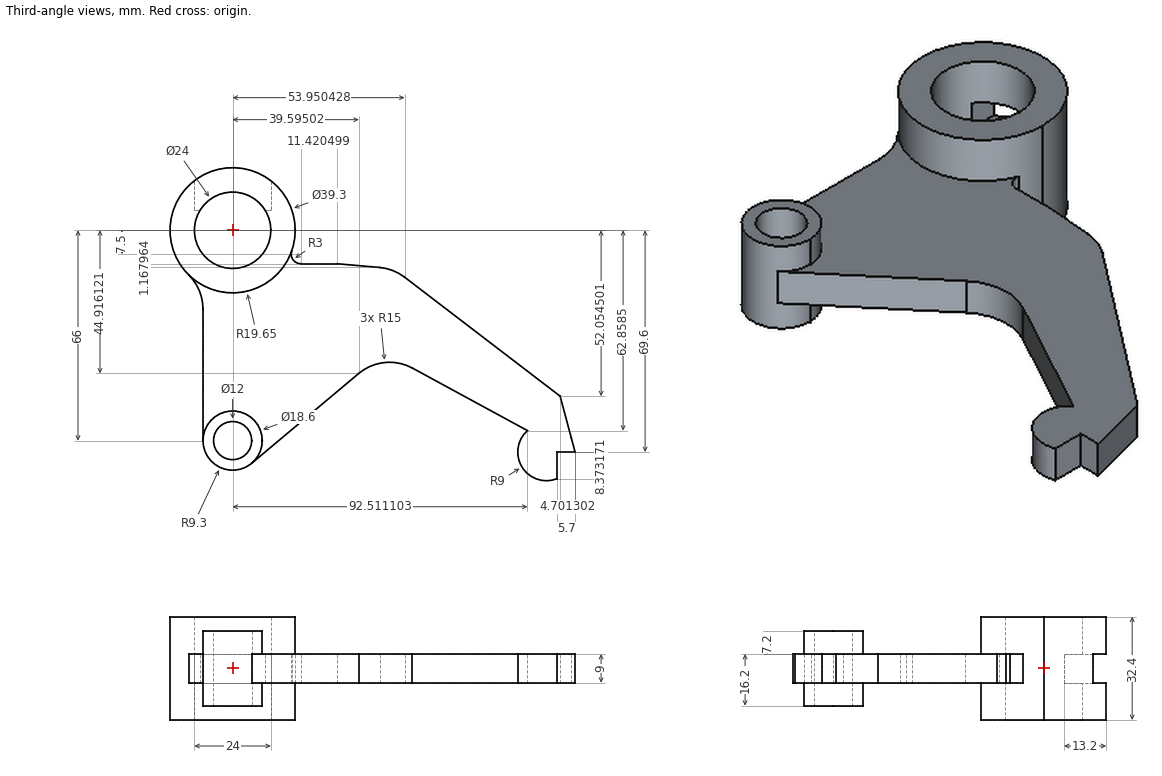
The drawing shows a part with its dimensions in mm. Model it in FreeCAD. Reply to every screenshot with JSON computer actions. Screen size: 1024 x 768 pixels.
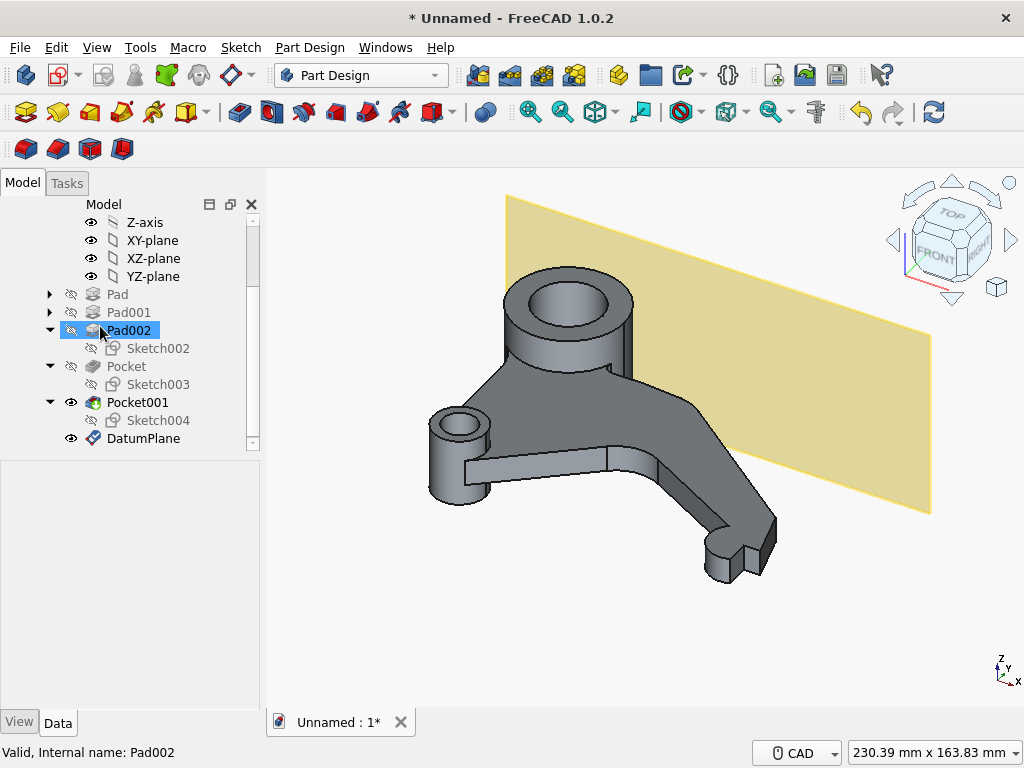
{"action": "left_click", "coordinate": [116, 438]}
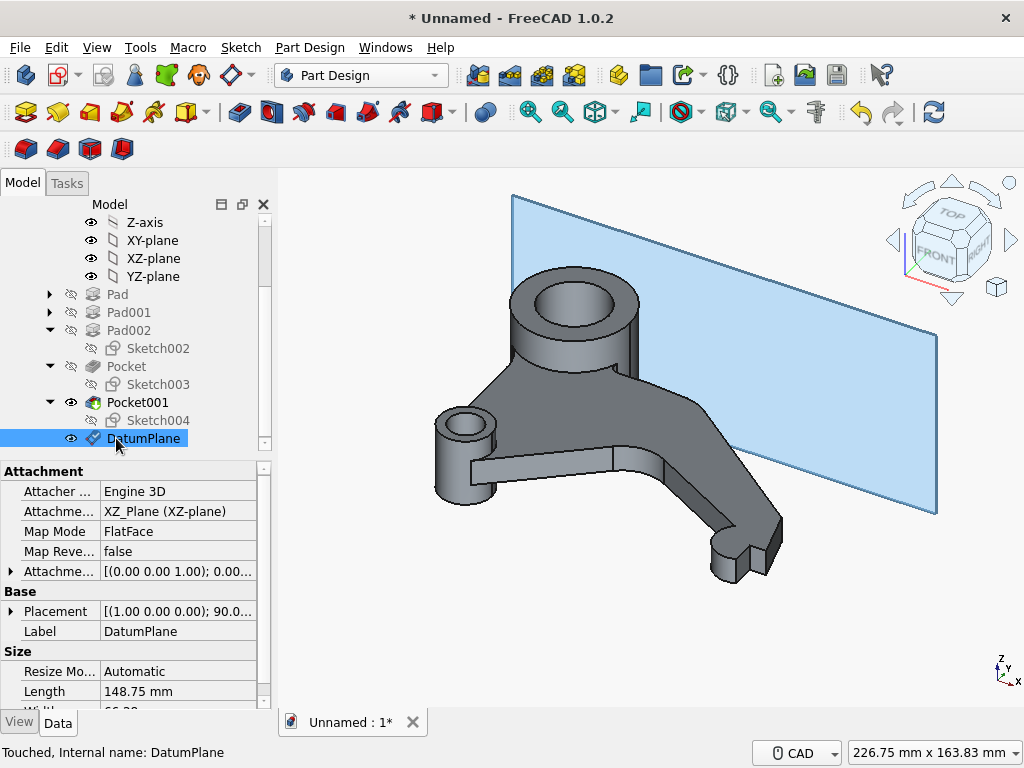
{"action": "left_click", "coordinate": [58, 76]}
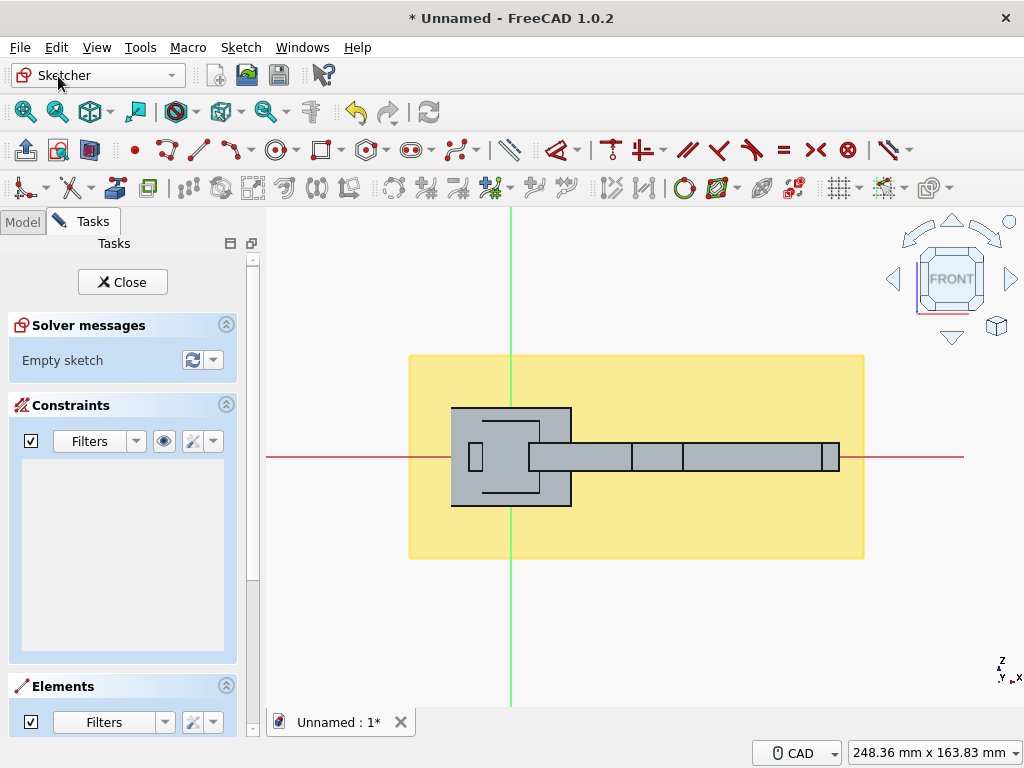
{"action": "key", "text": "q s"}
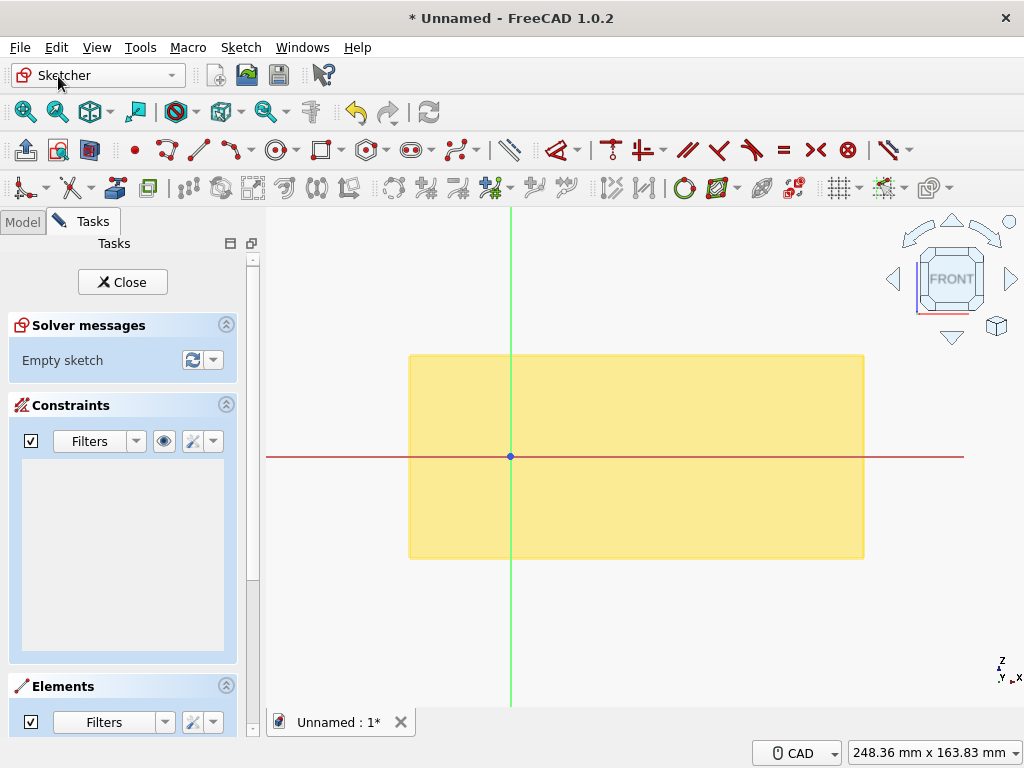
{"action": "scroll", "coordinate": [494, 457], "scroll_direction": "up", "scroll_amount": 8}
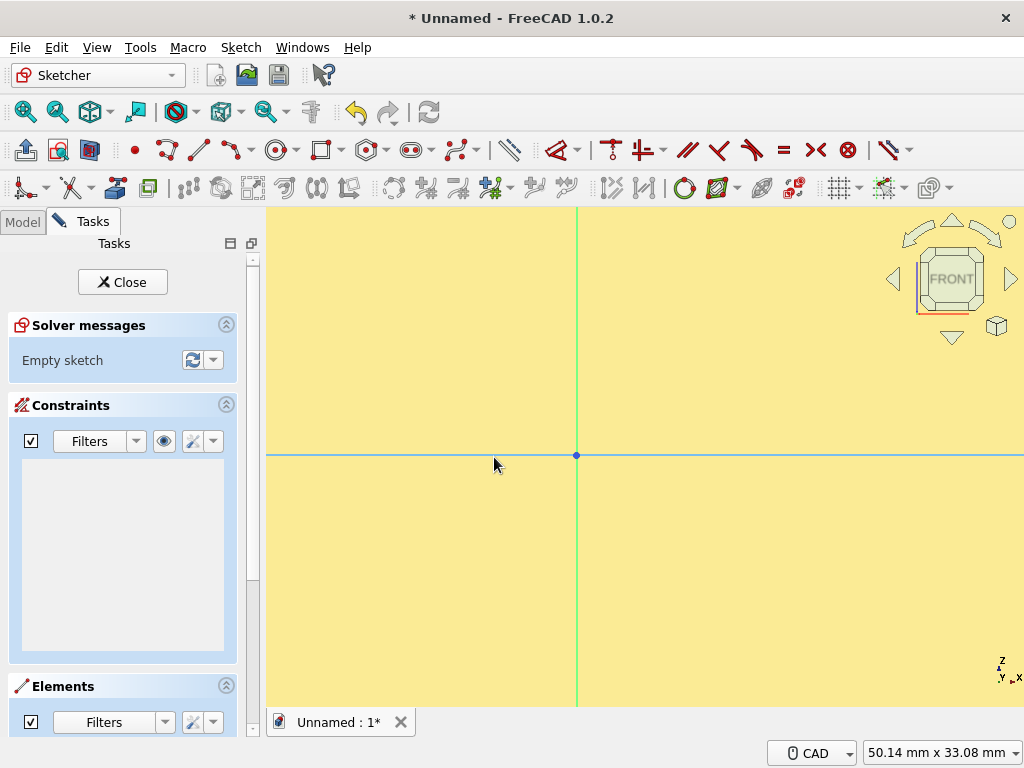
{"action": "key", "text": "g v"}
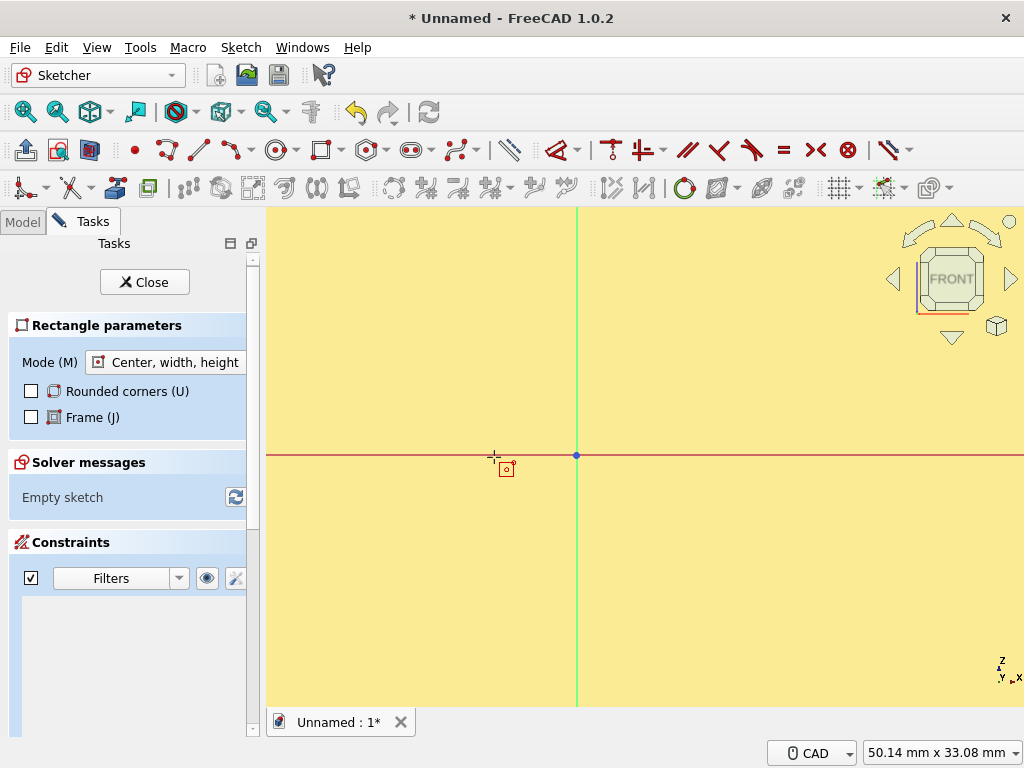
{"action": "left_click", "coordinate": [577, 455]}
{"action": "mouse_move", "coordinate": [758, 387]}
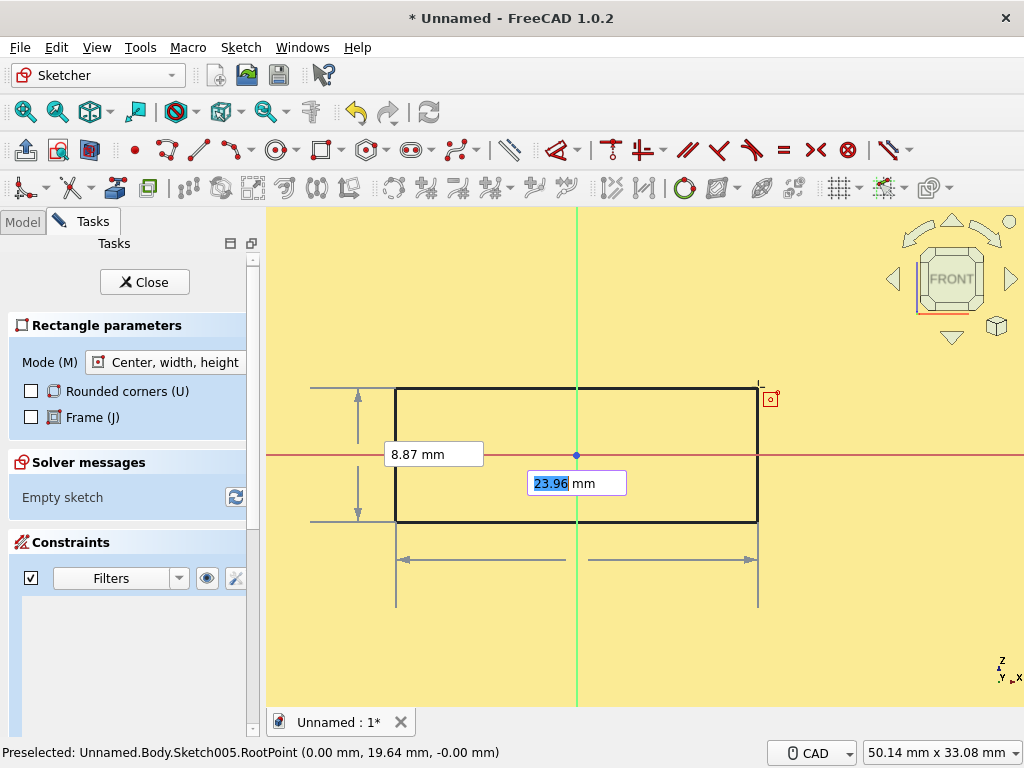
{"action": "type", "text": "24"}
{"action": "key", "text": "Tab"}
{"action": "type", "text": "9"}
{"action": "key", "text": "Return"}
{"action": "key", "text": "Escape"}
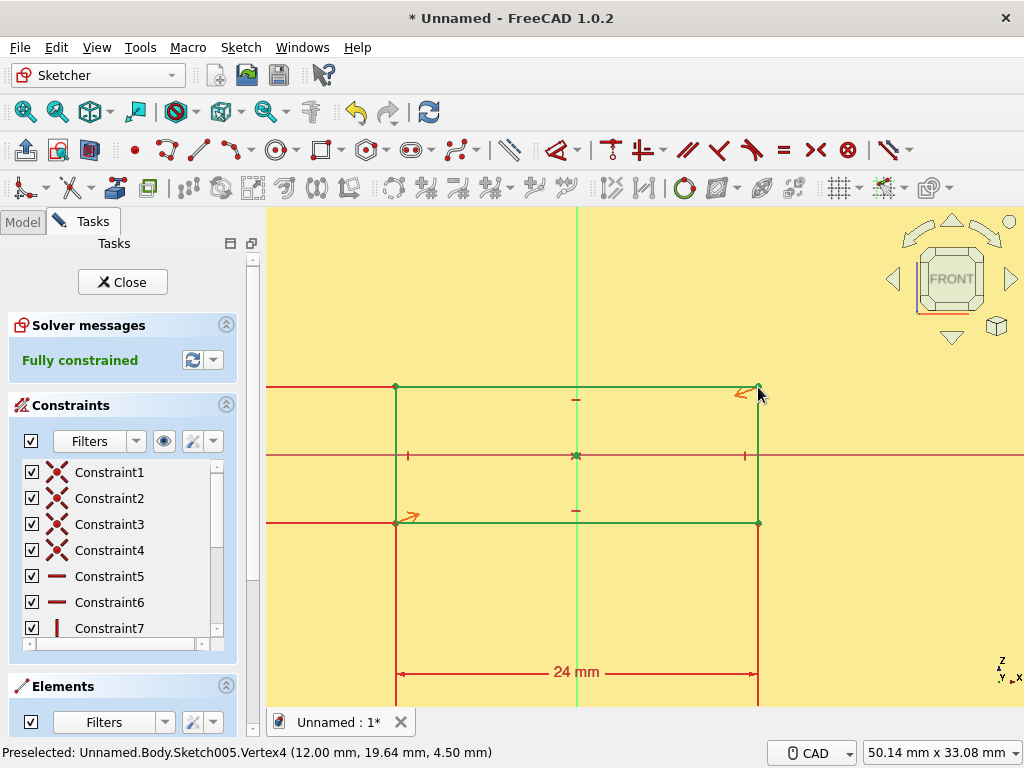
{"action": "left_click", "coordinate": [123, 282]}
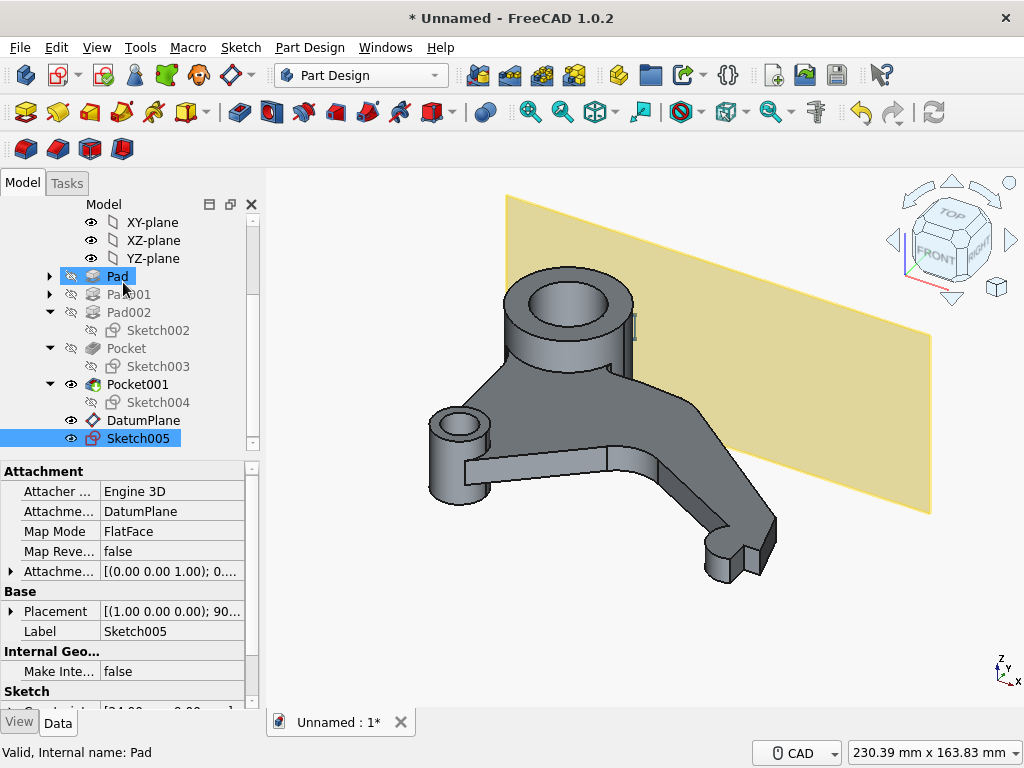
{"action": "left_click", "coordinate": [240, 112]}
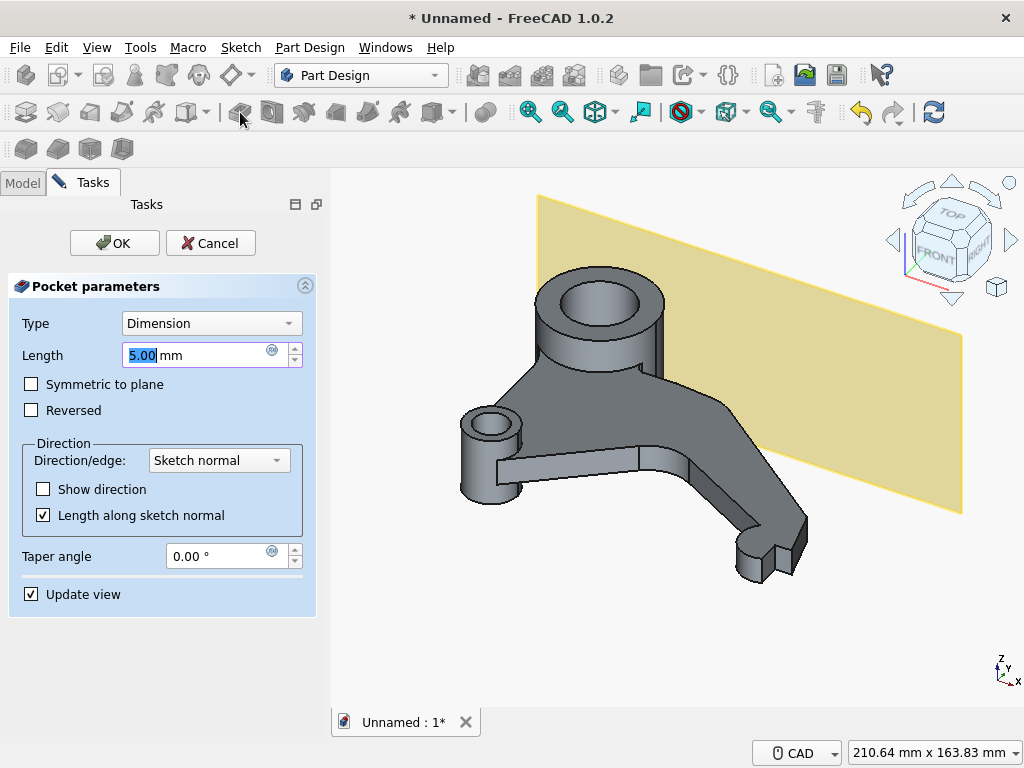
{"action": "type", "text": "13.2"}
{"action": "key", "text": "Tab"}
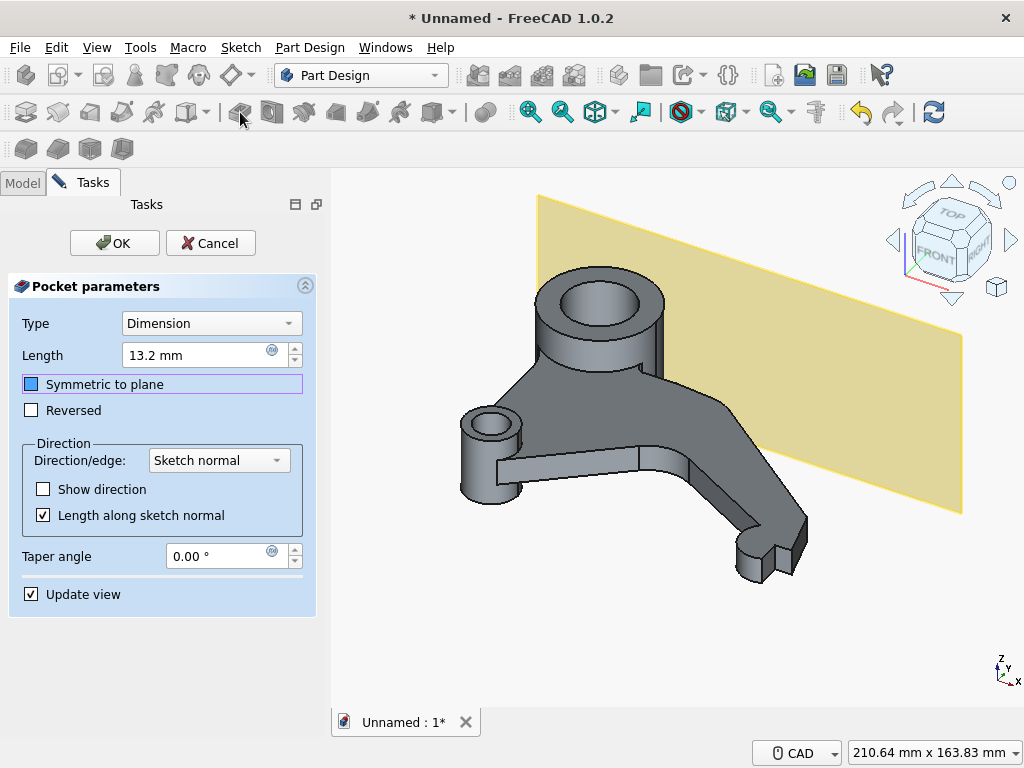
{"action": "left_click", "coordinate": [30, 410]}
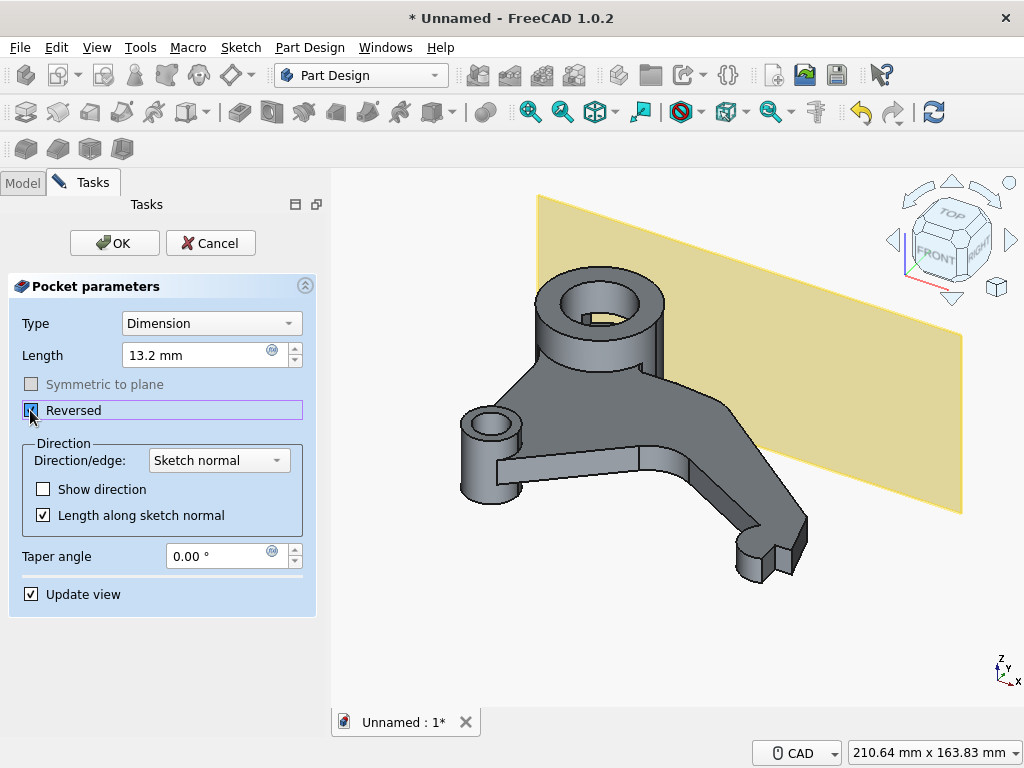
{"action": "left_click", "coordinate": [115, 243]}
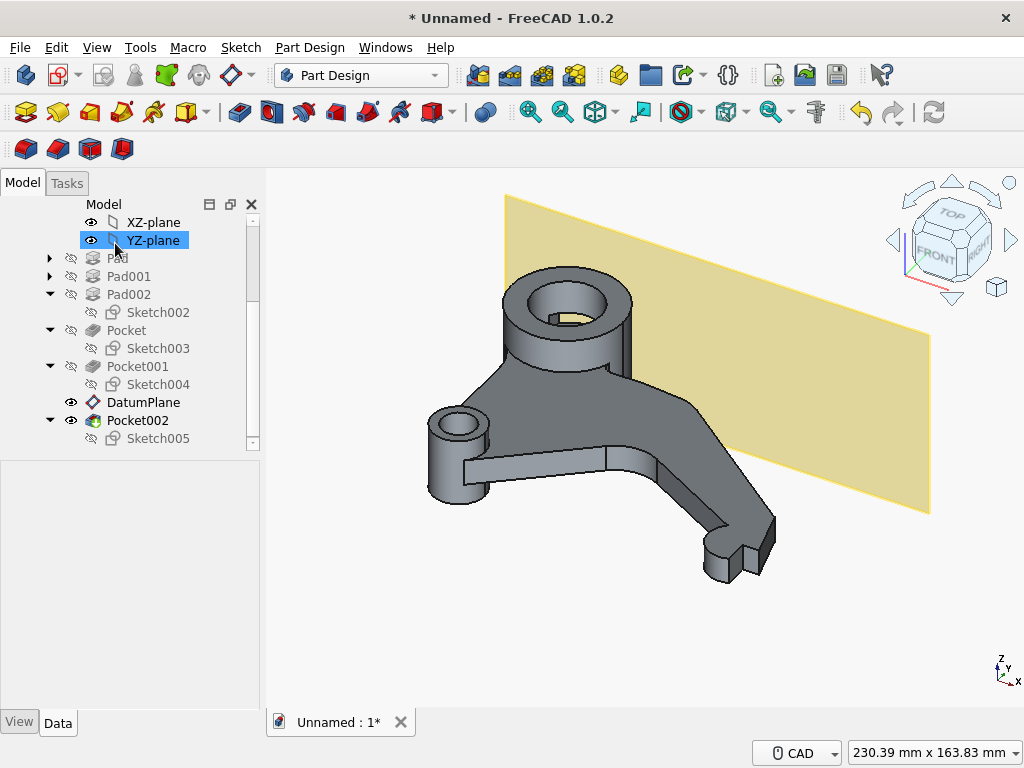
{"action": "left_click", "coordinate": [116, 402]}
{"action": "key", "text": "space"}